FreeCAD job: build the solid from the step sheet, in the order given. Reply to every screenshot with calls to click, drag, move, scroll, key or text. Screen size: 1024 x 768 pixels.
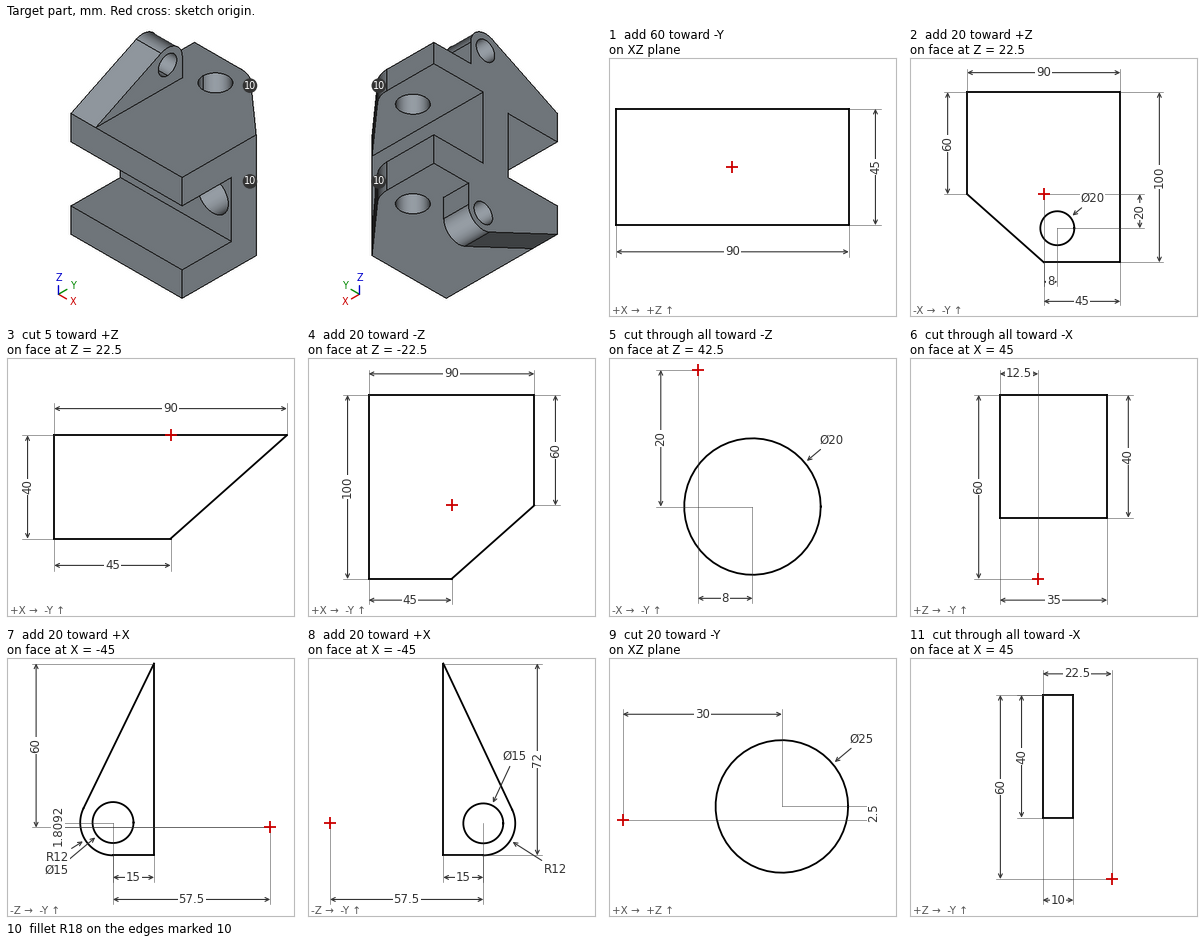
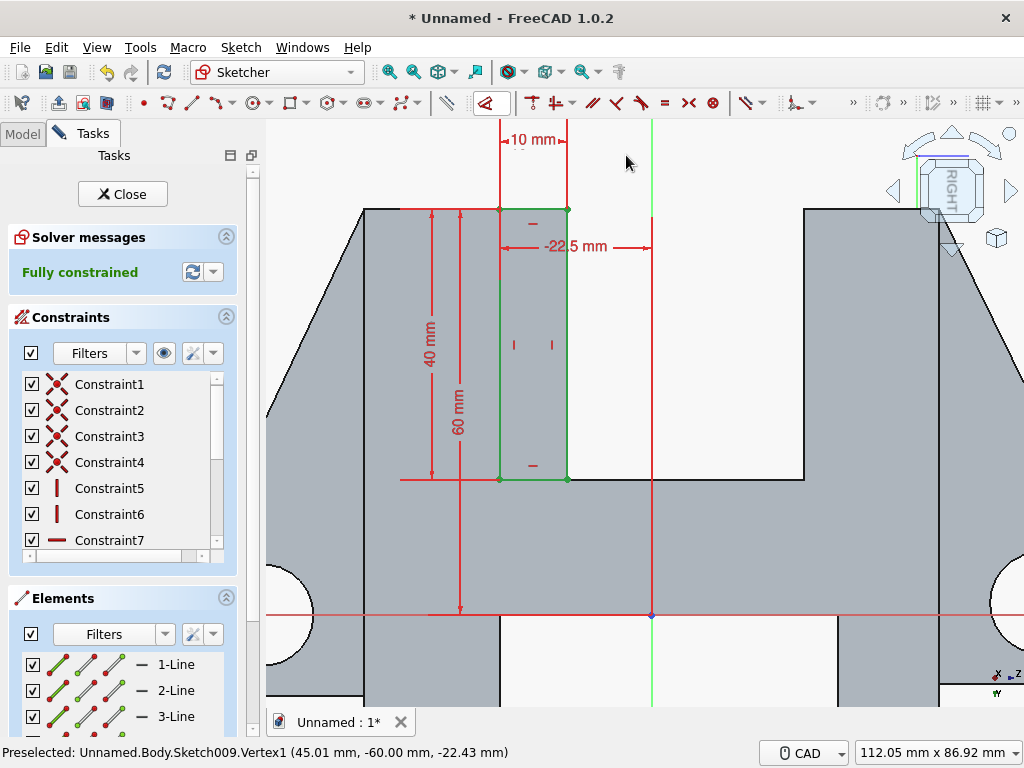
click(123, 194)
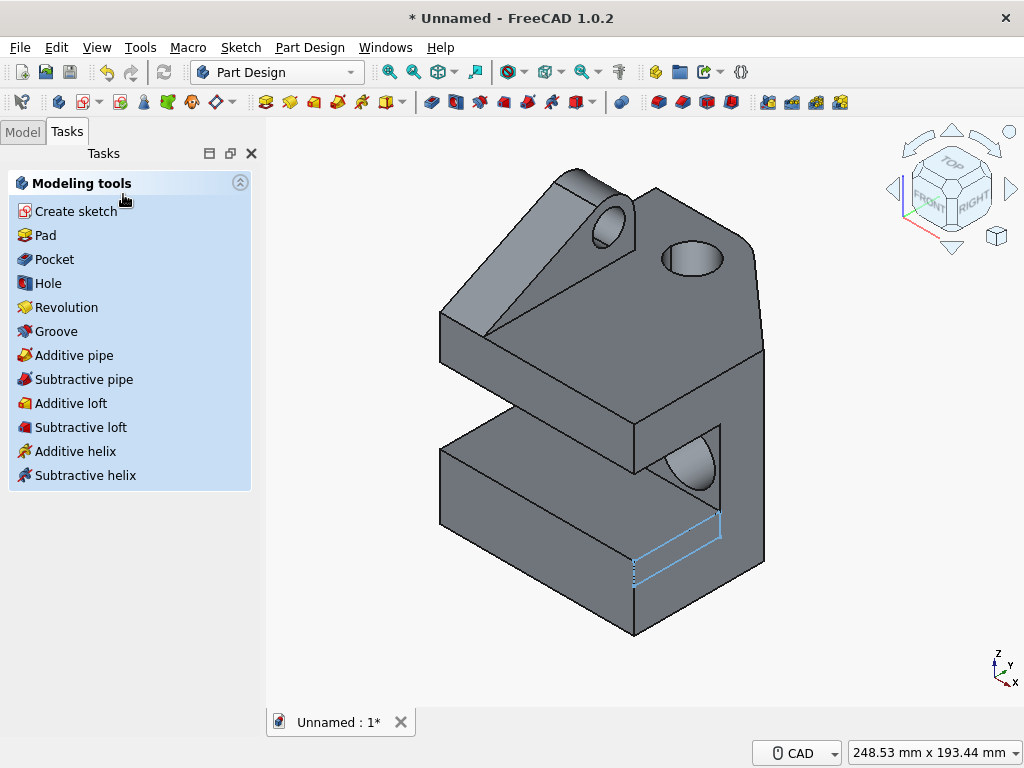
click(432, 102)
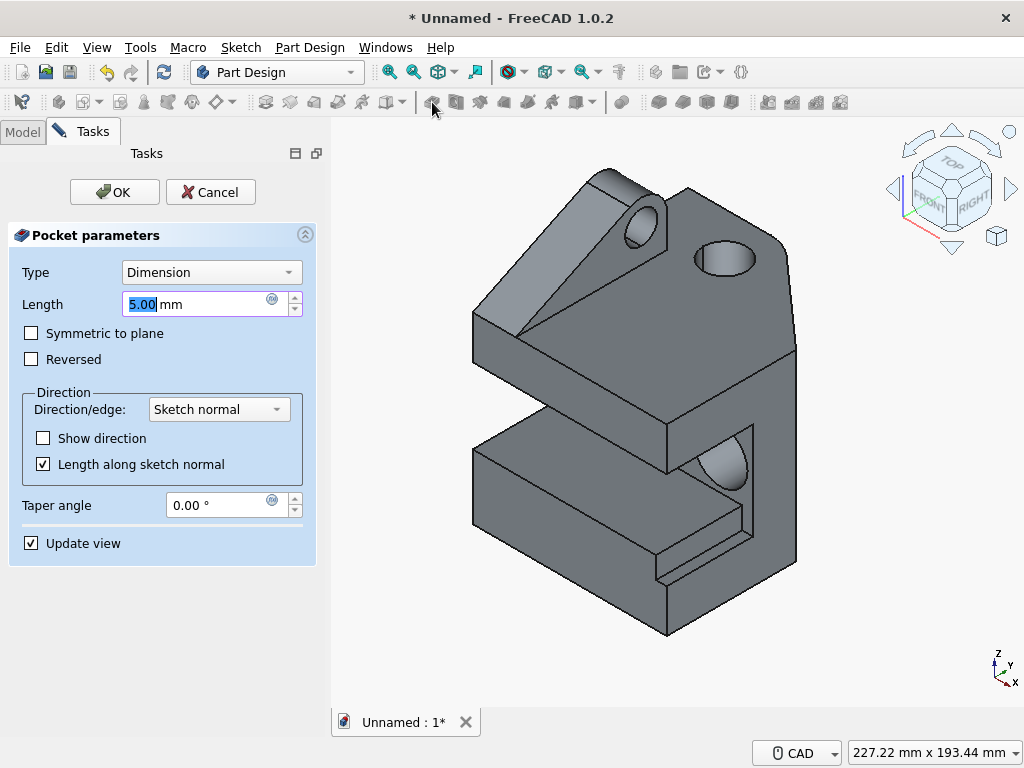
click(212, 272)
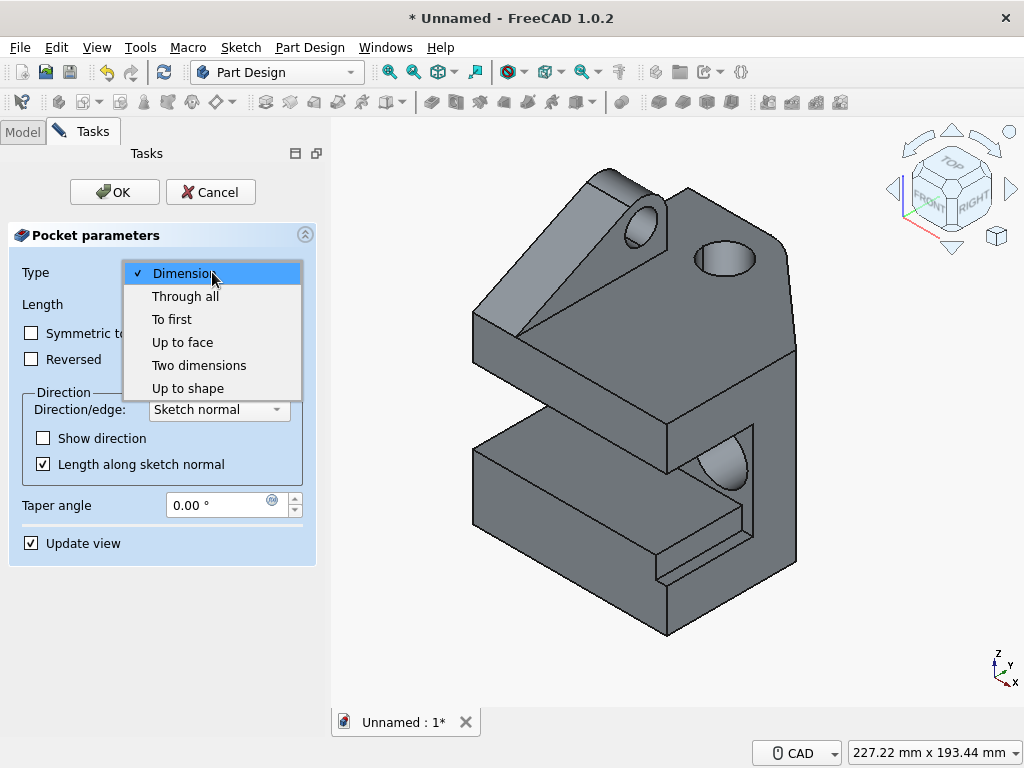
click(212, 296)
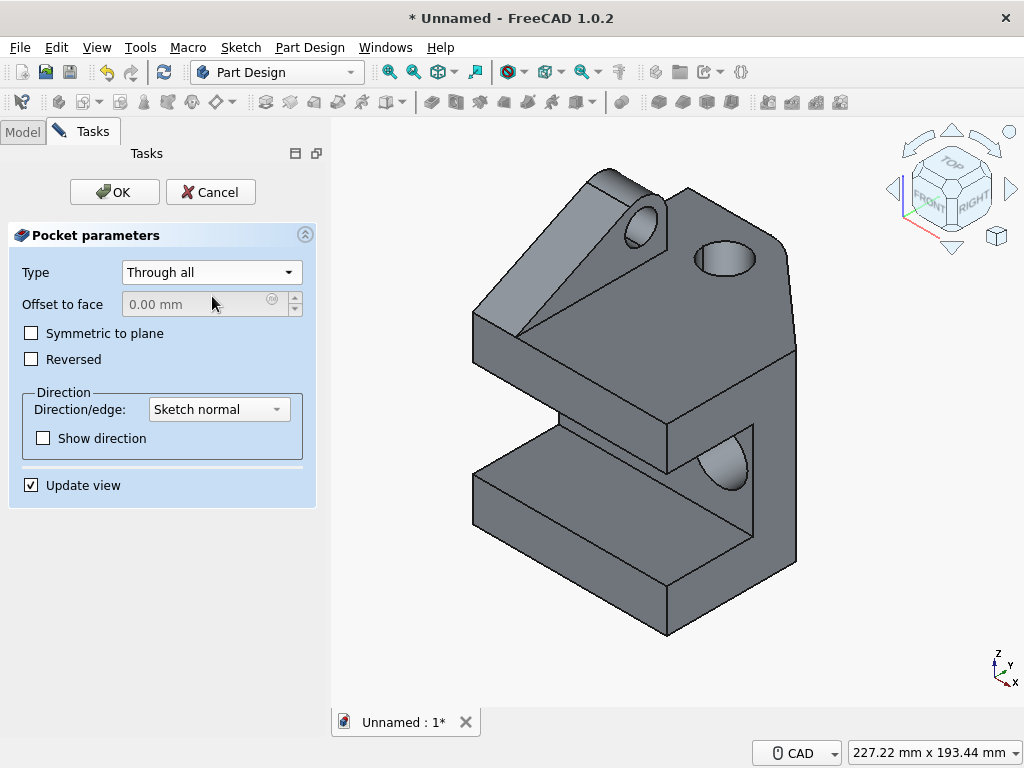
click(115, 192)